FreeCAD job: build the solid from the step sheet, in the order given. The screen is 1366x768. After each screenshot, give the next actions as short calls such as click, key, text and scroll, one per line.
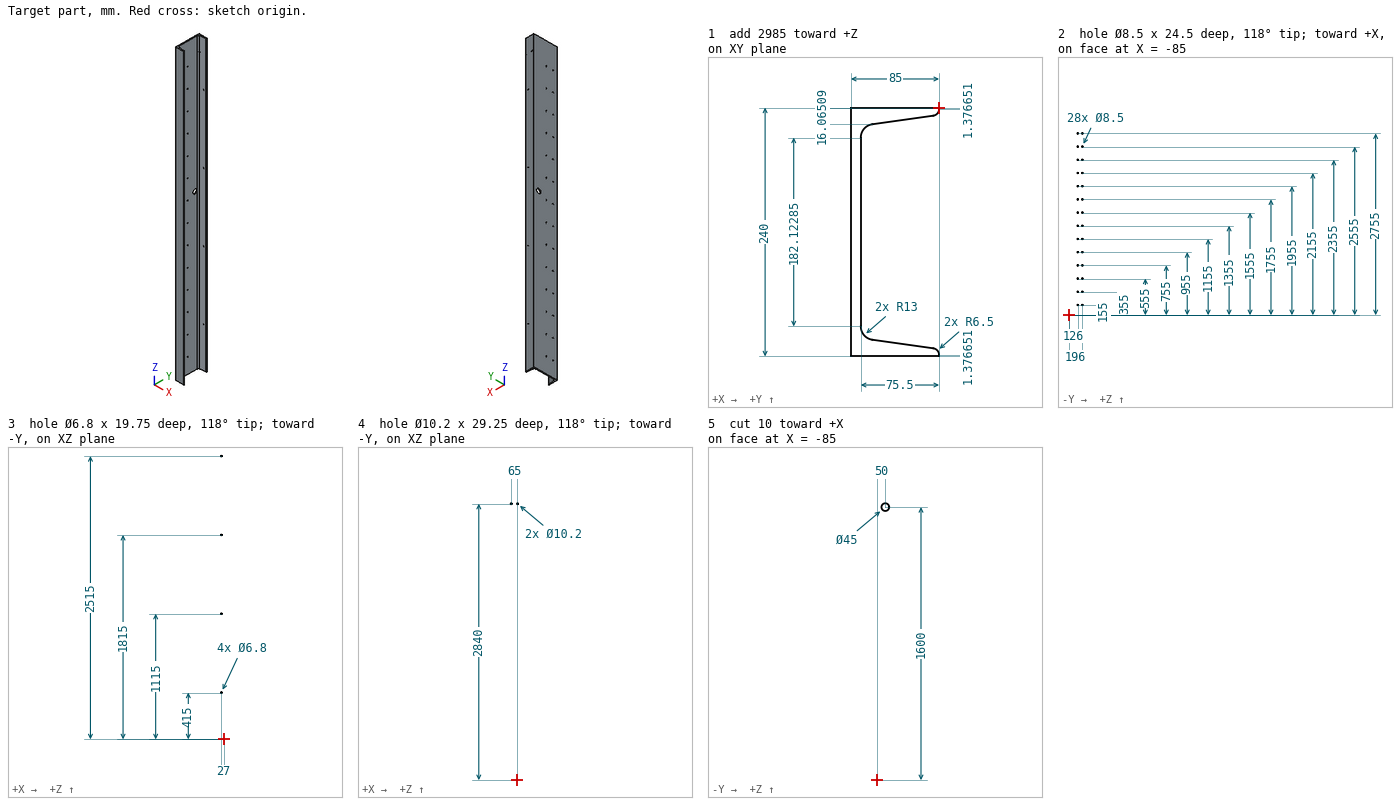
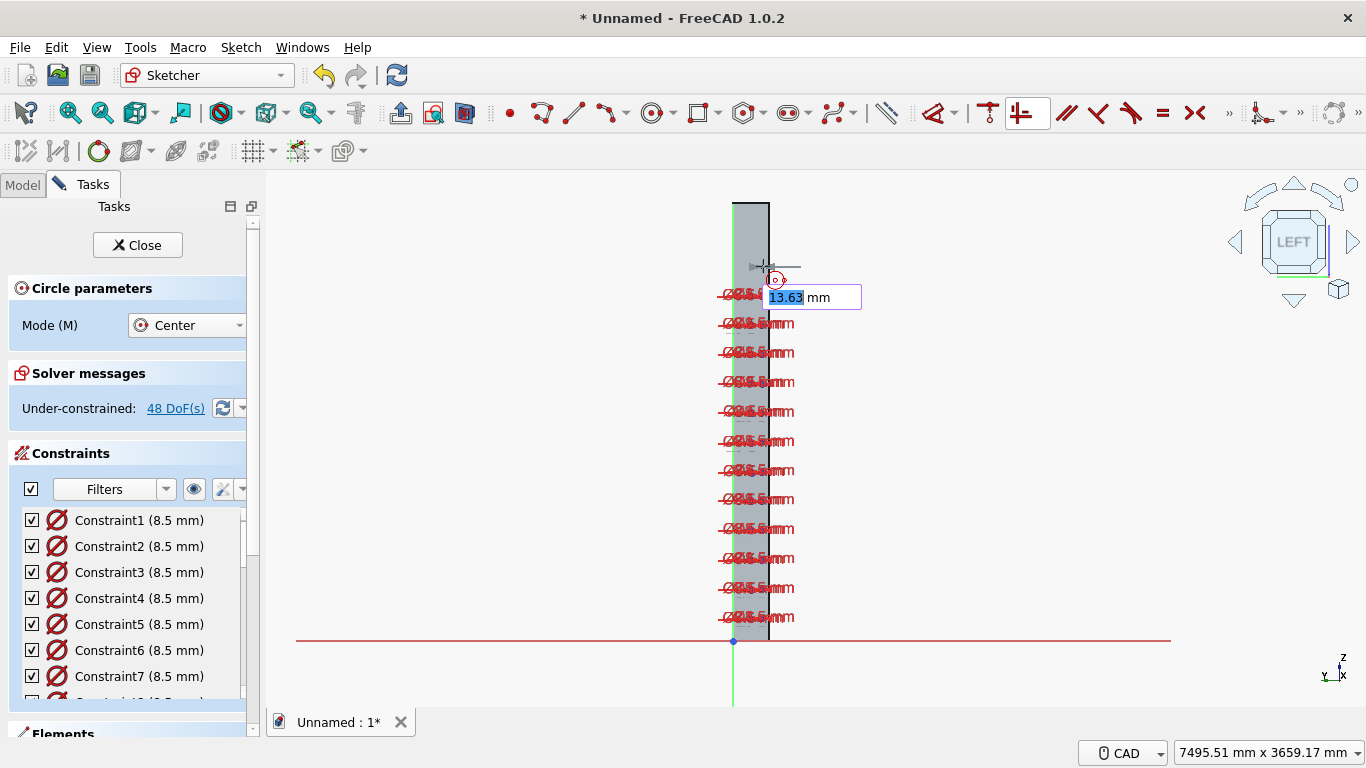
text(8.5)
key(Return)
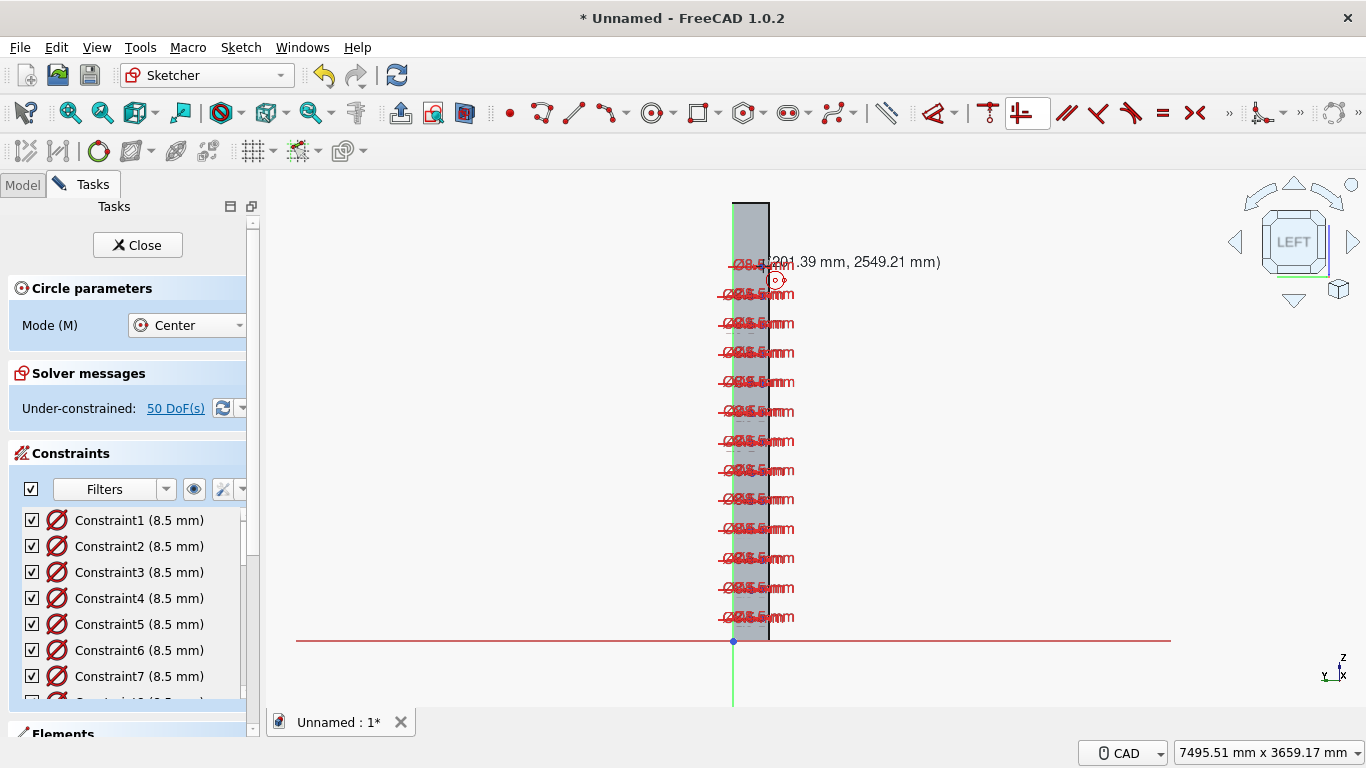
scroll(752, 266, up, 18)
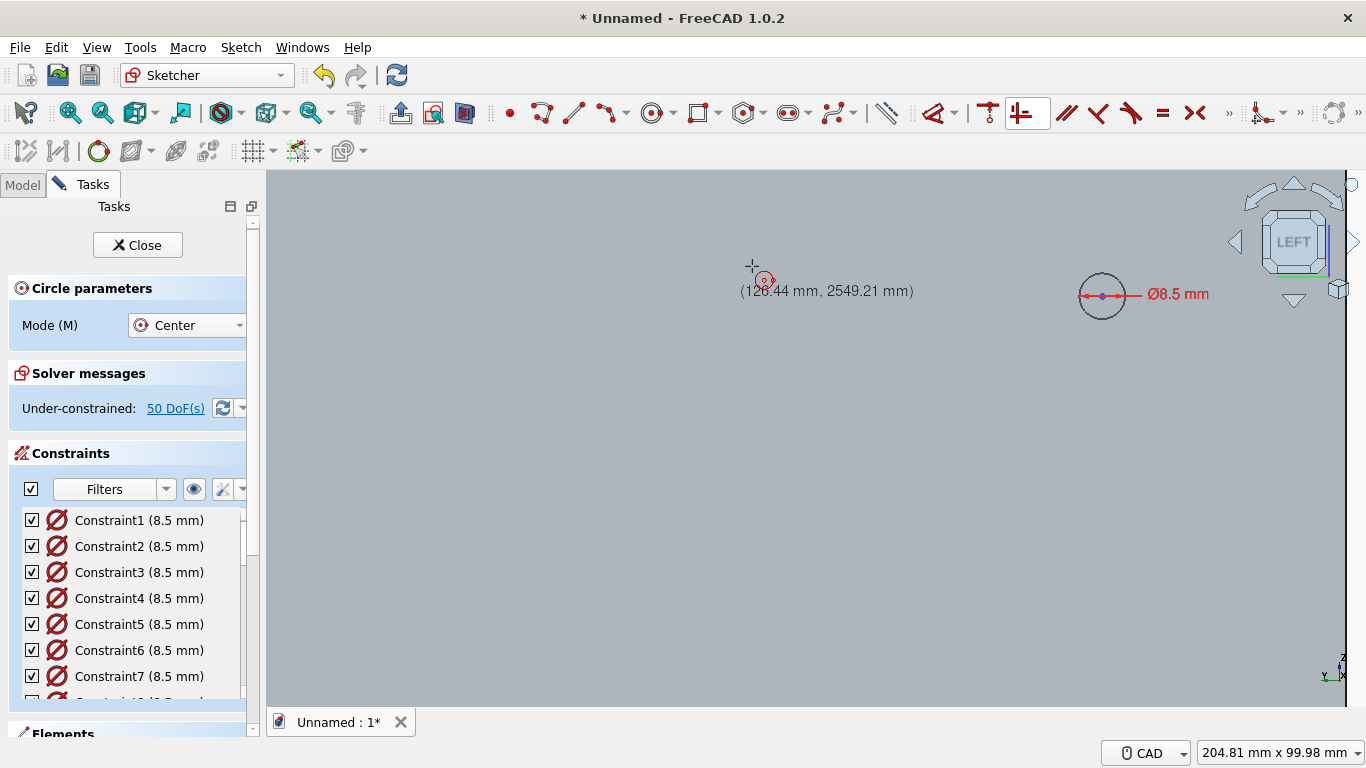
scroll(752, 266, down, 18)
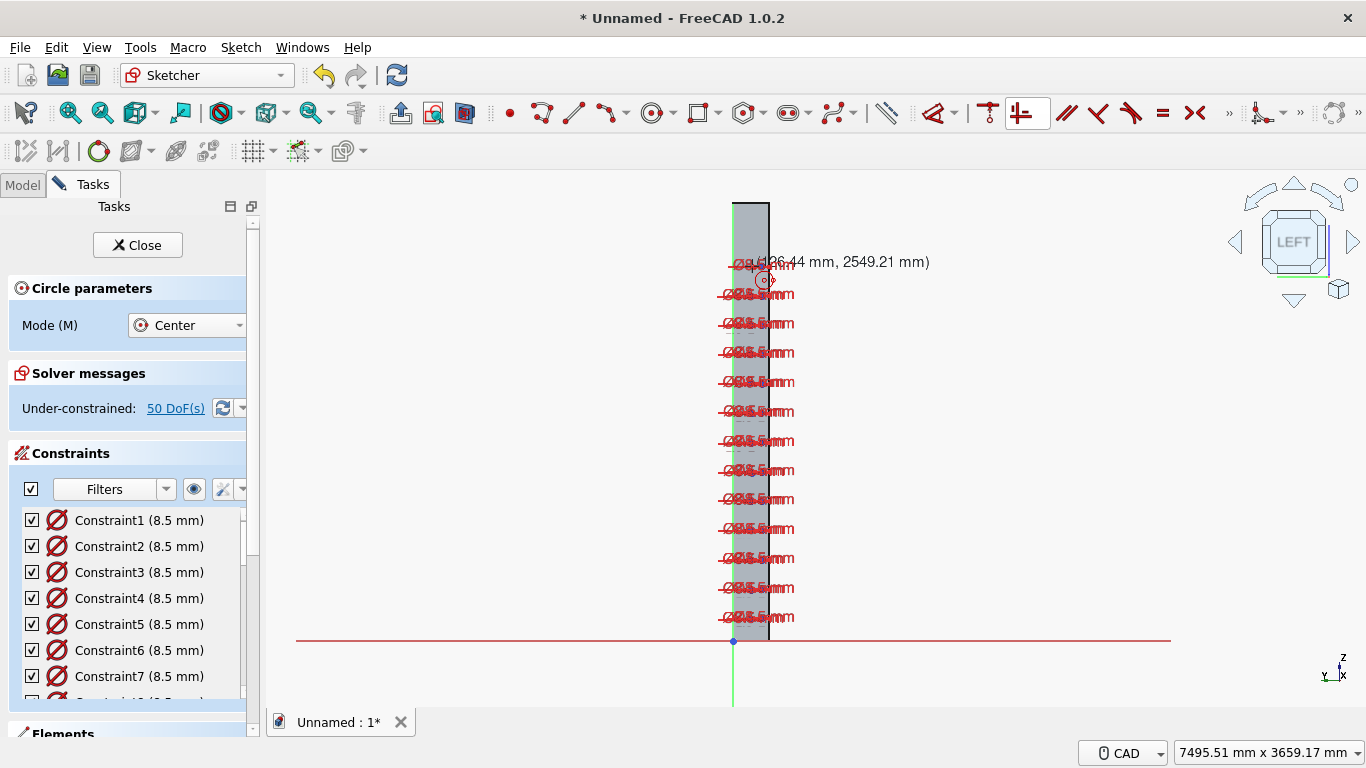
scroll(752, 266, up, 3)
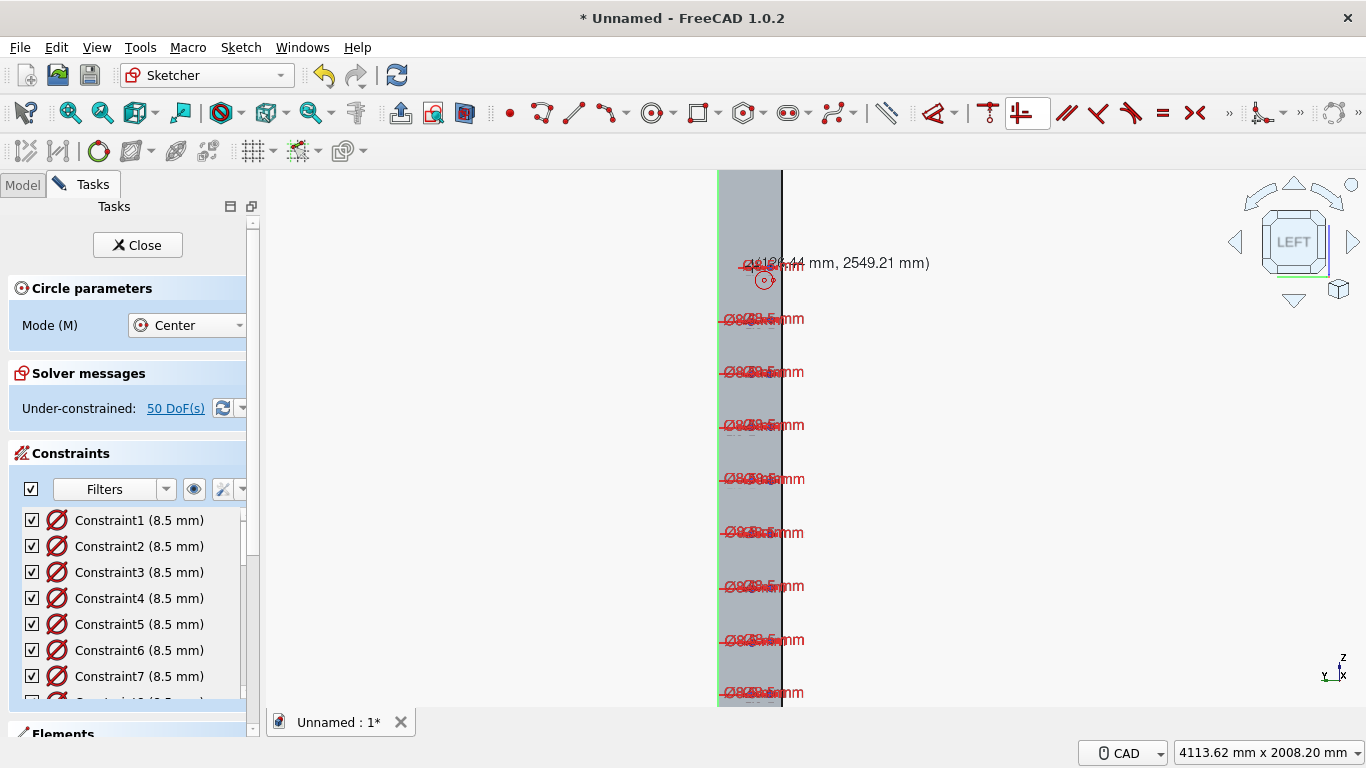
click(752, 266)
move(752, 265)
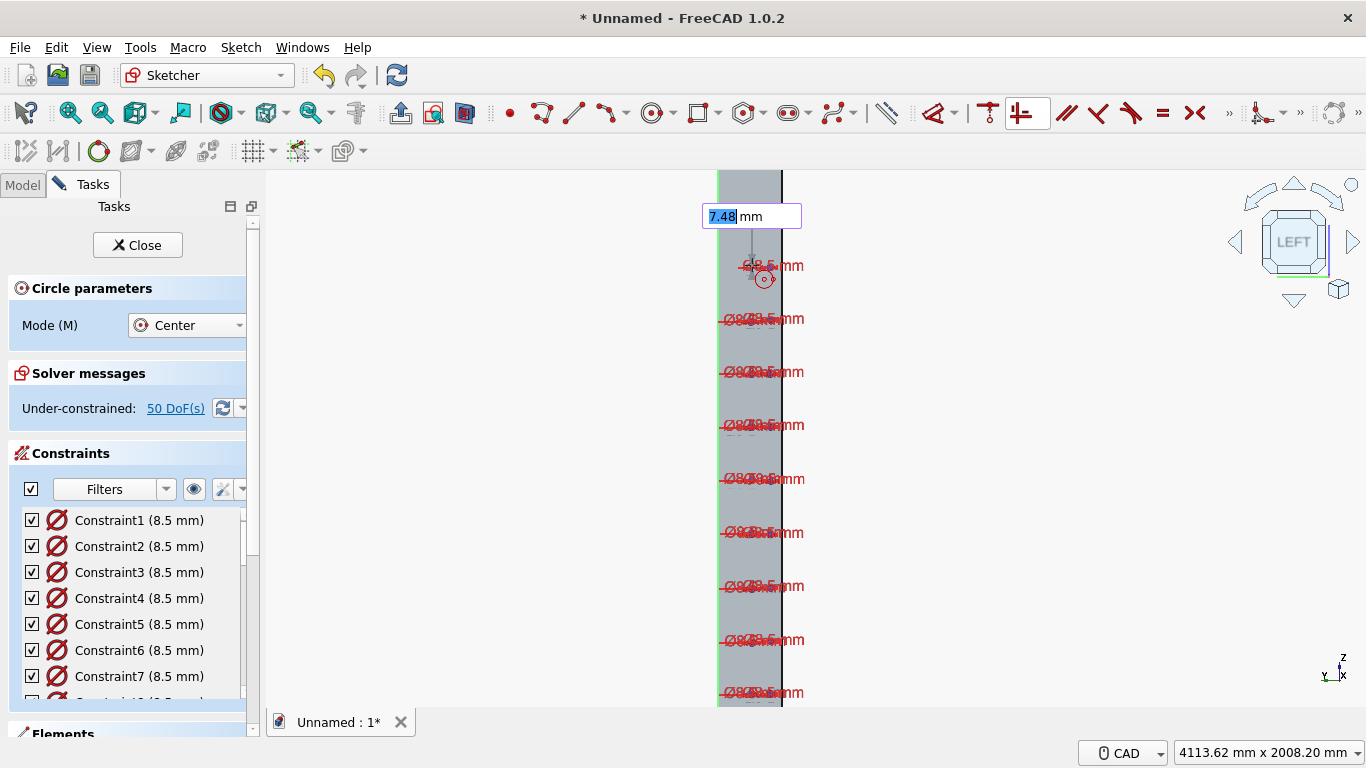
text(8.5)
key(Return)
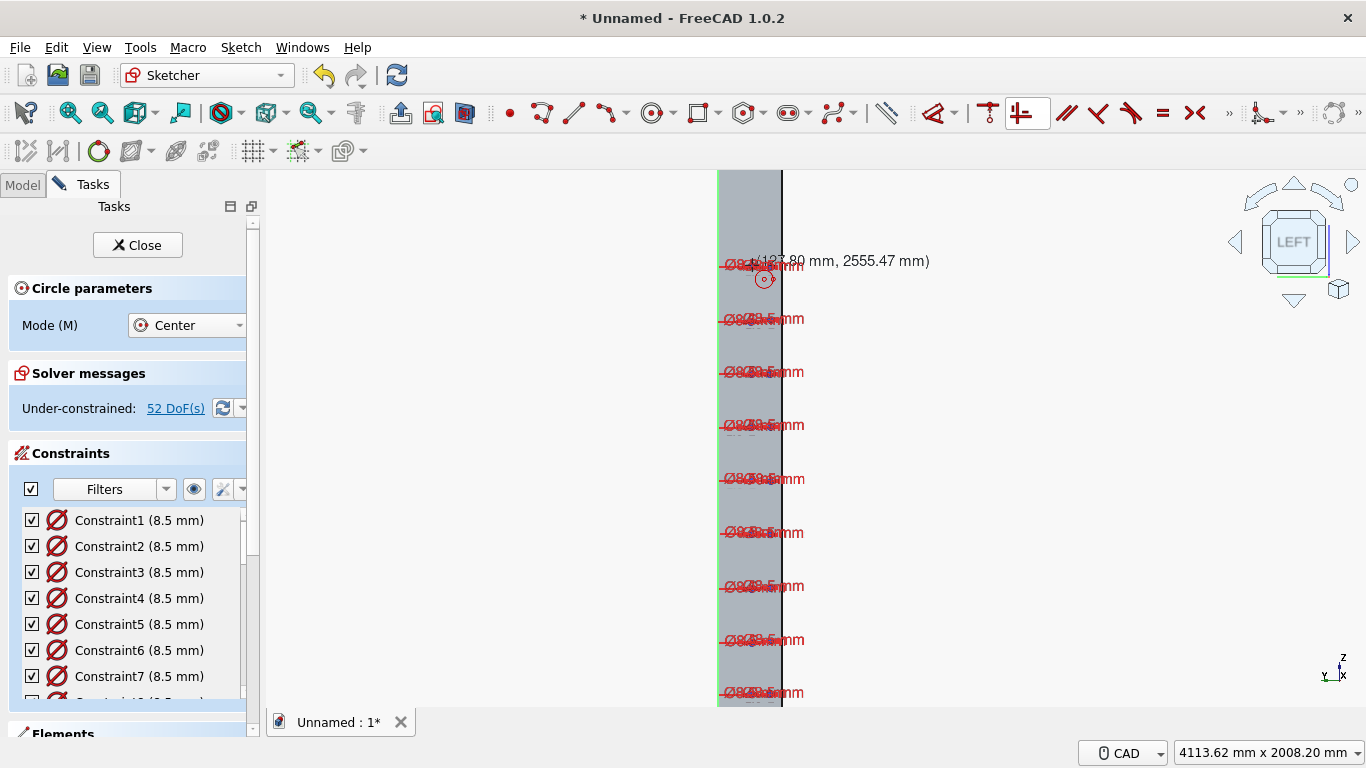
scroll(752, 213, up, 15)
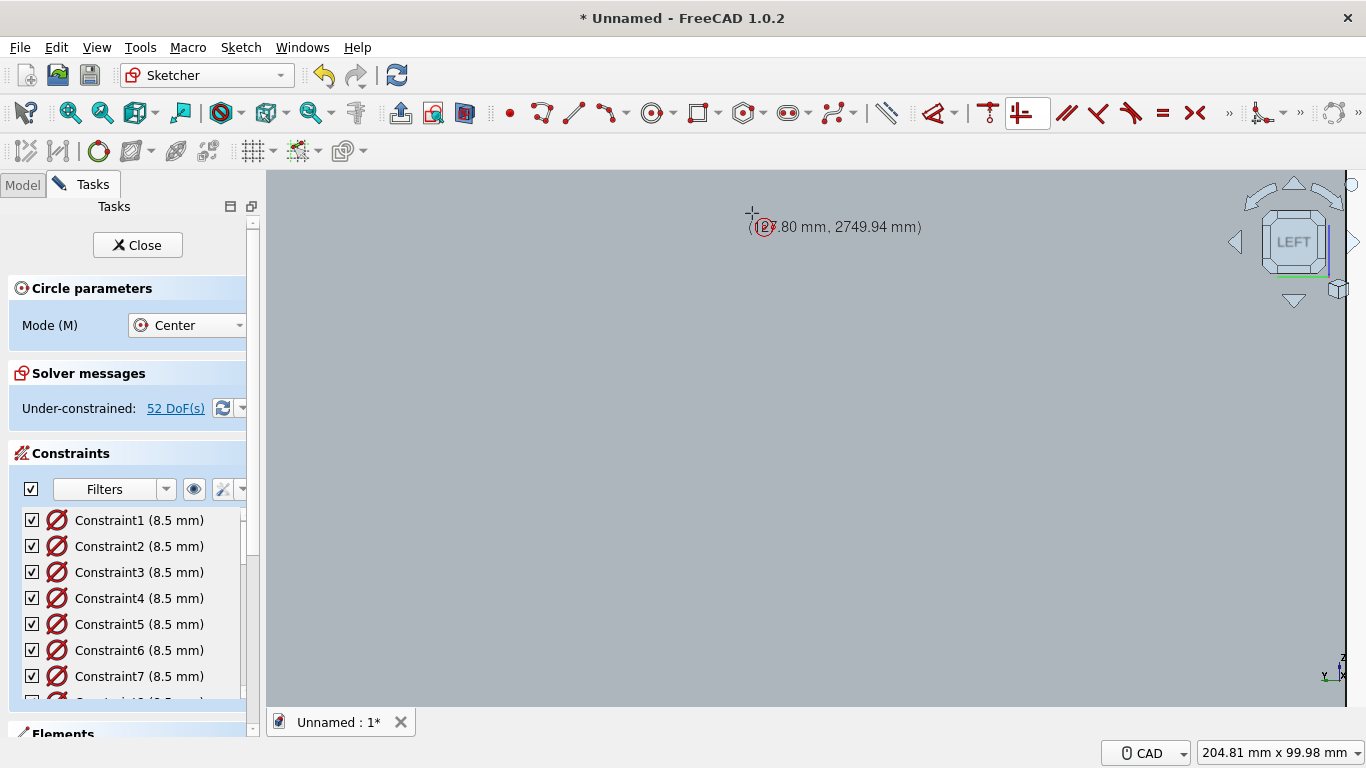
scroll(752, 238, down, 18)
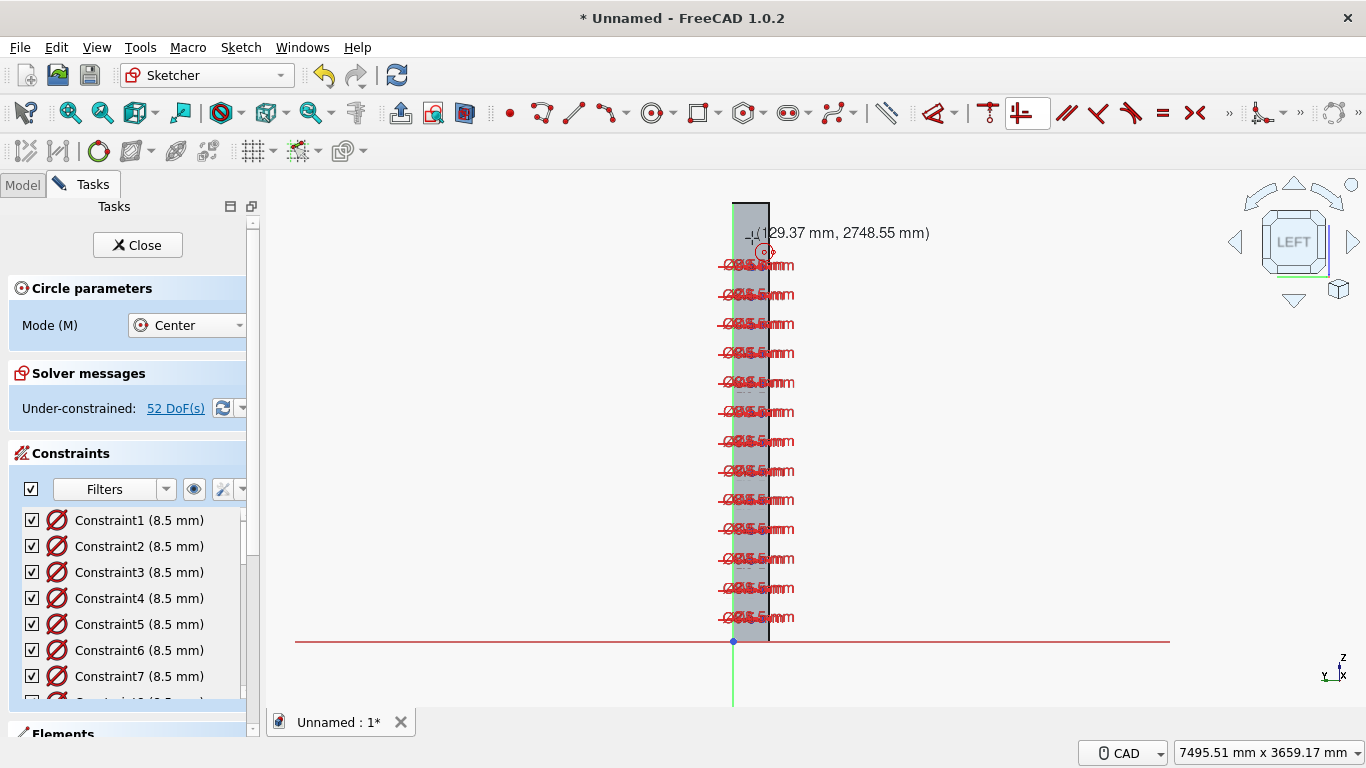
click(752, 237)
move(752, 237)